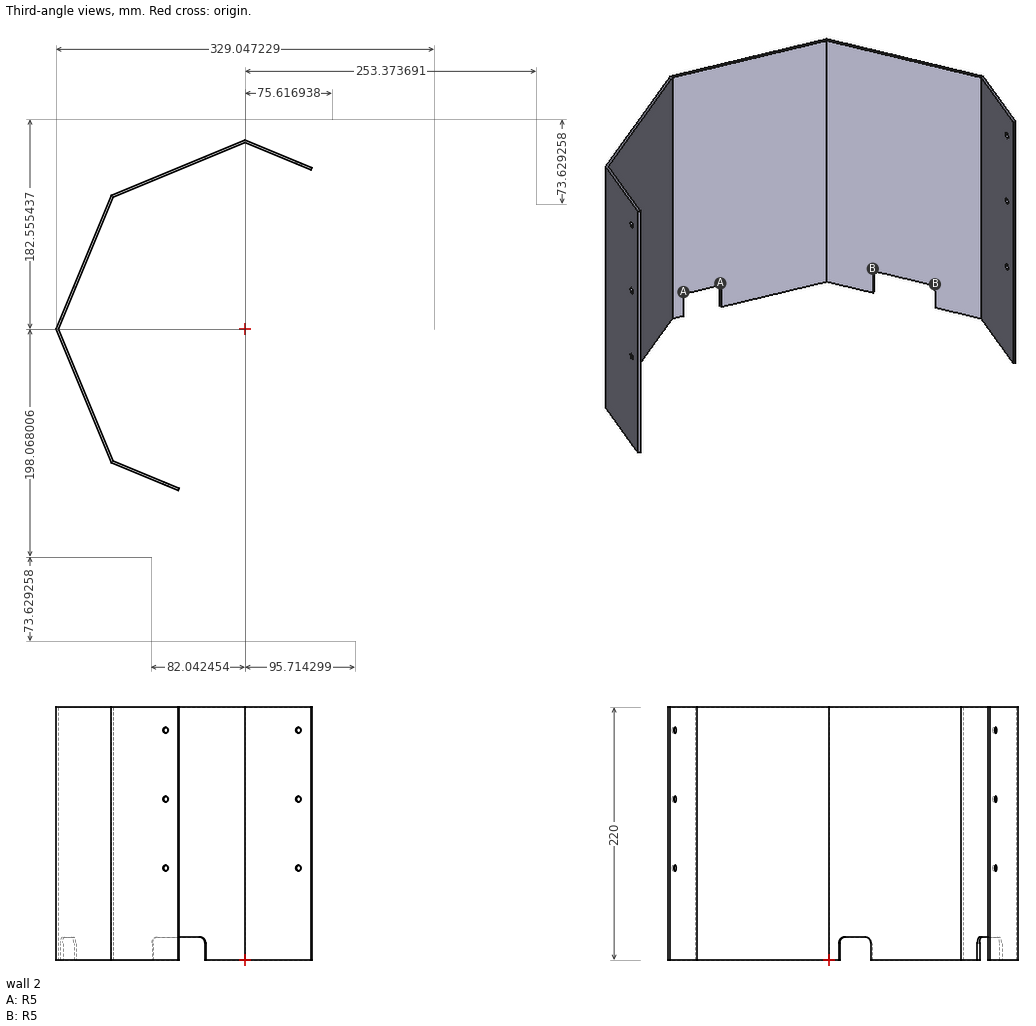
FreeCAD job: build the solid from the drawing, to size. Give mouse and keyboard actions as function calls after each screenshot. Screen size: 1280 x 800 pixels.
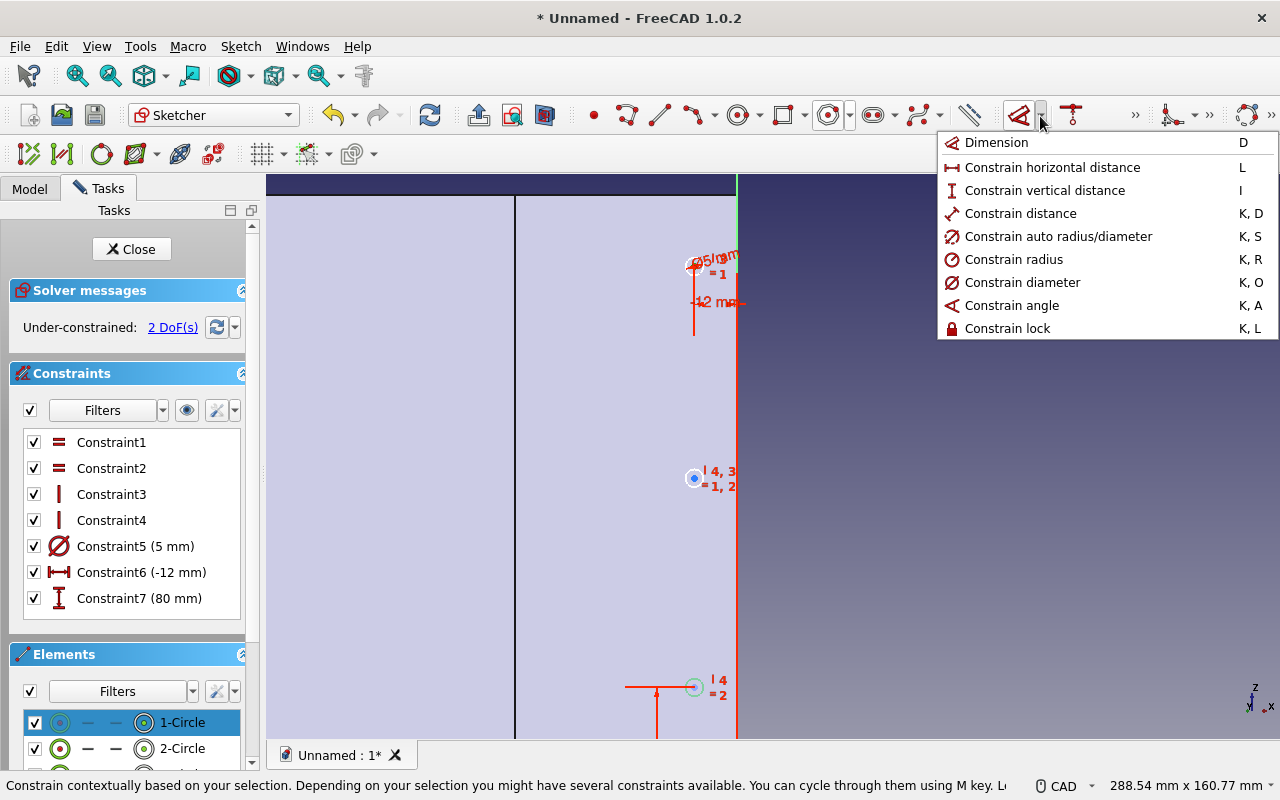
click(1108, 190)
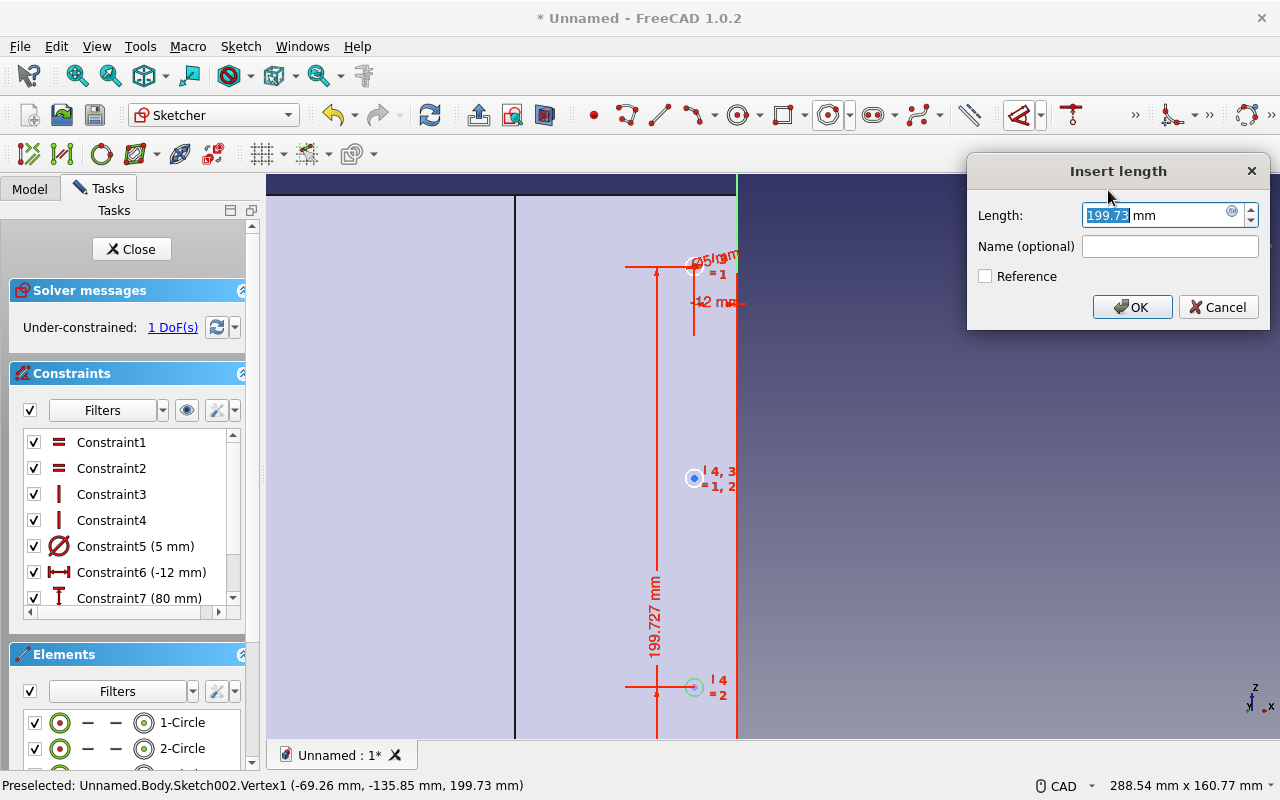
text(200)
key(Return)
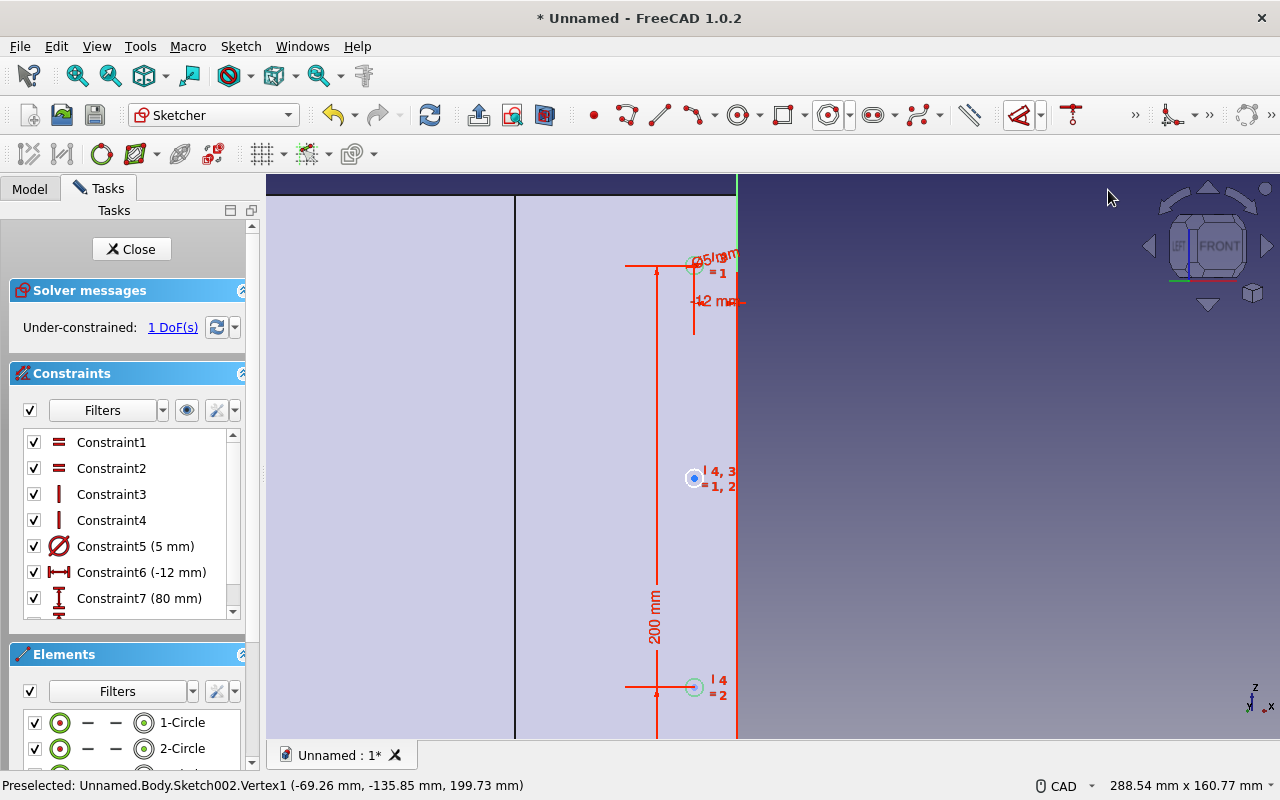
click(694, 478)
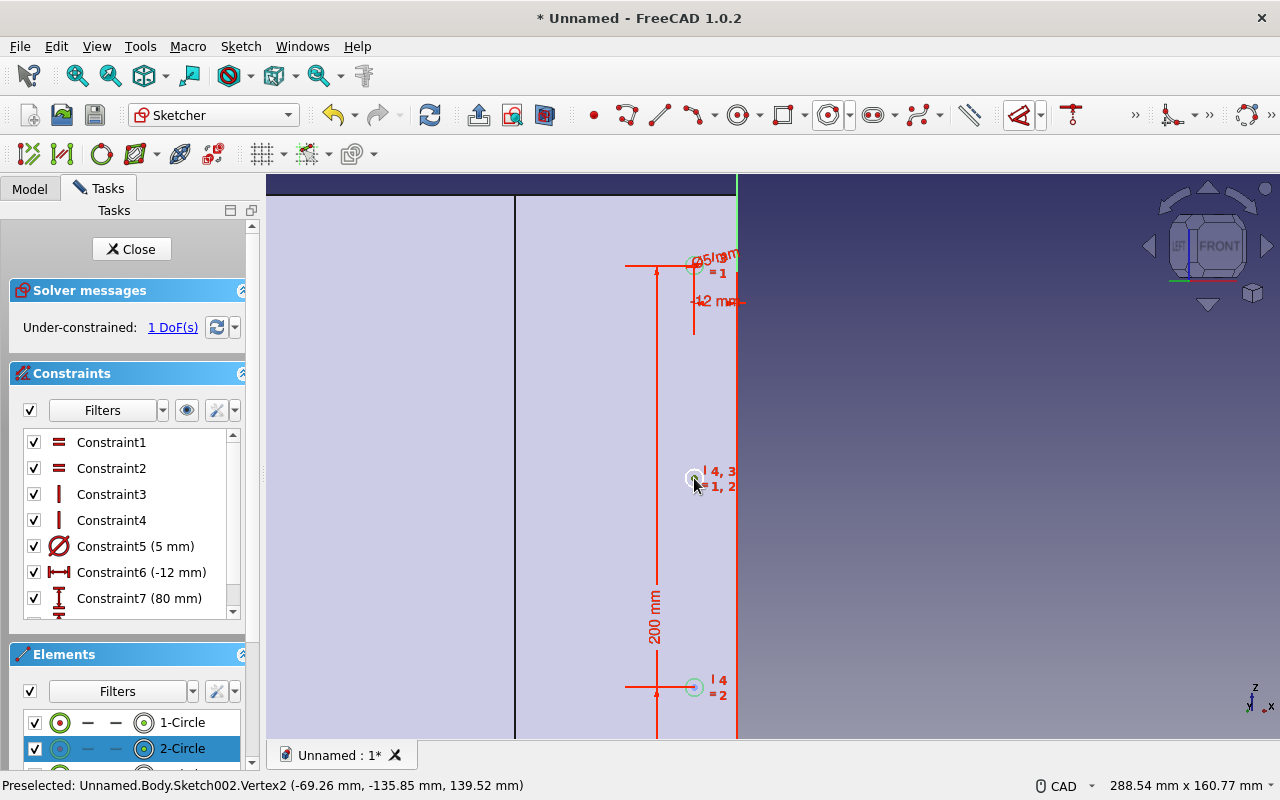
click(1040, 116)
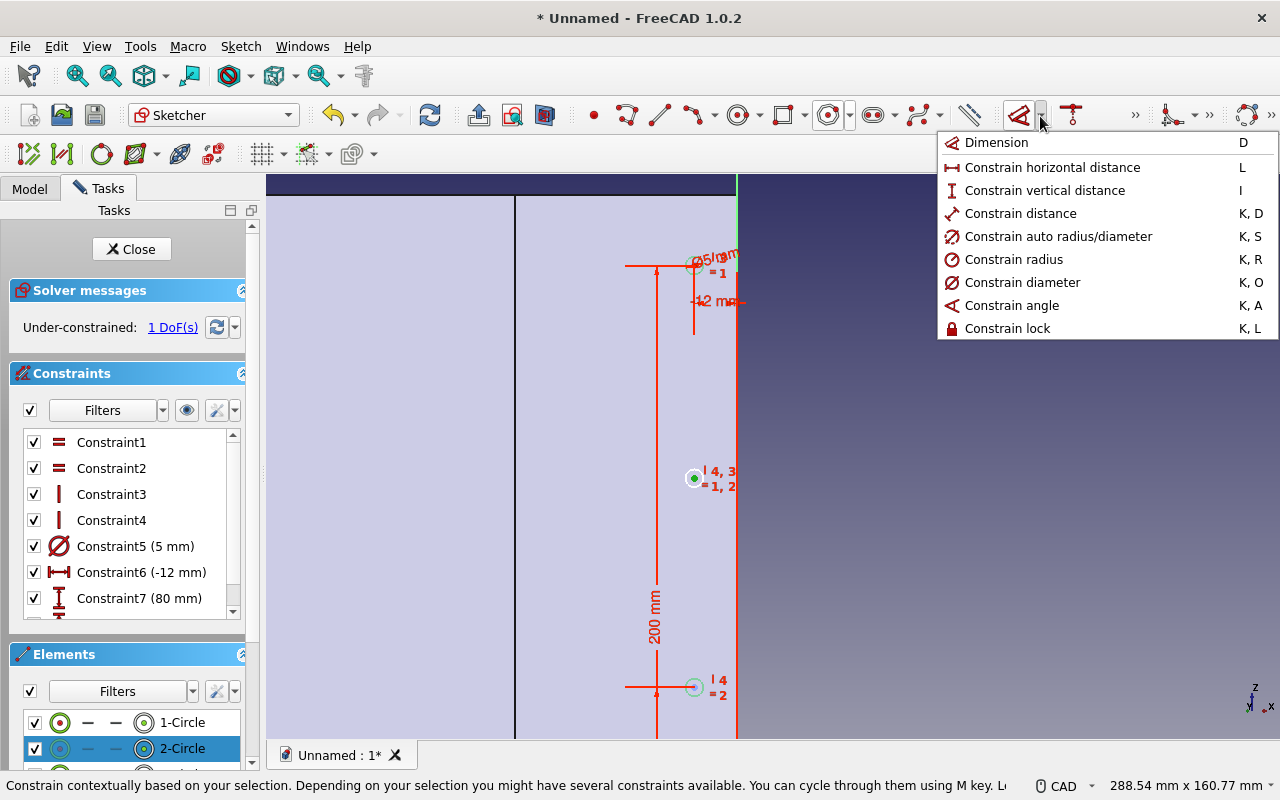
click(1108, 190)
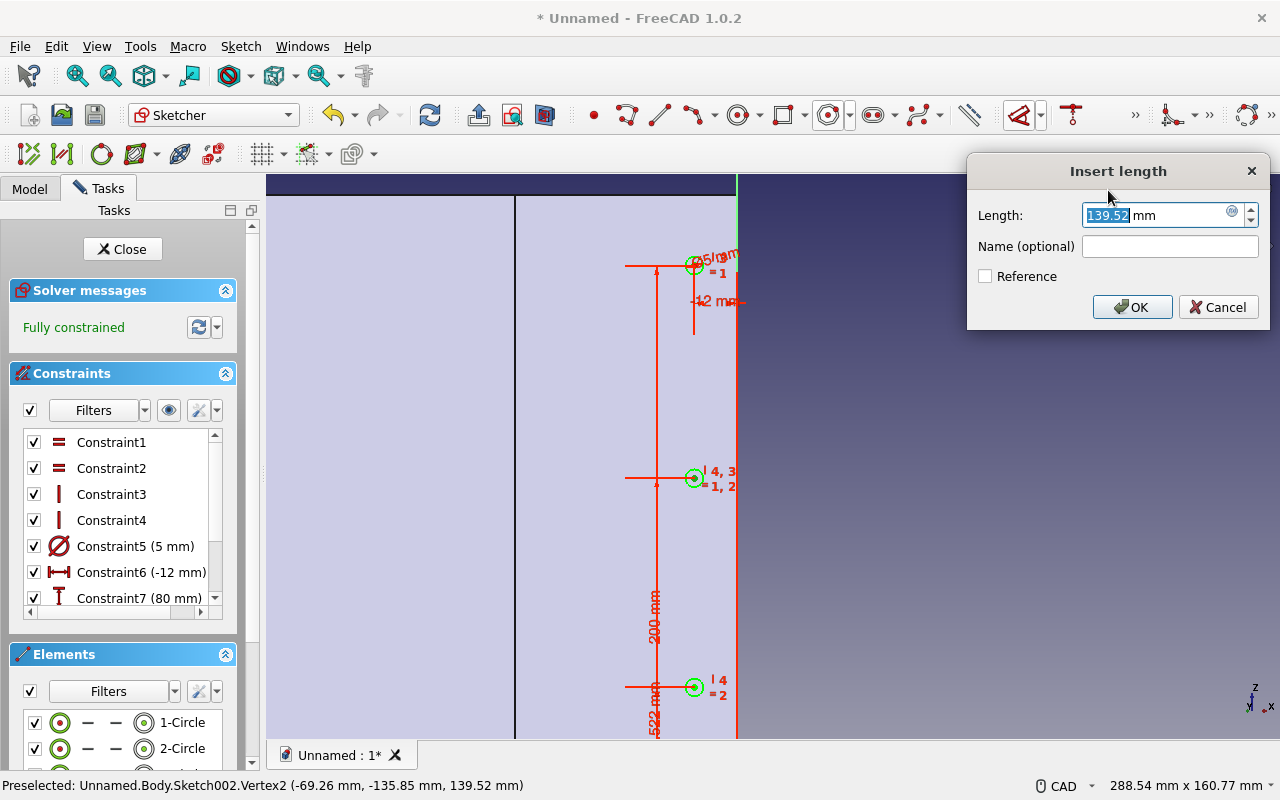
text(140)
key(Return)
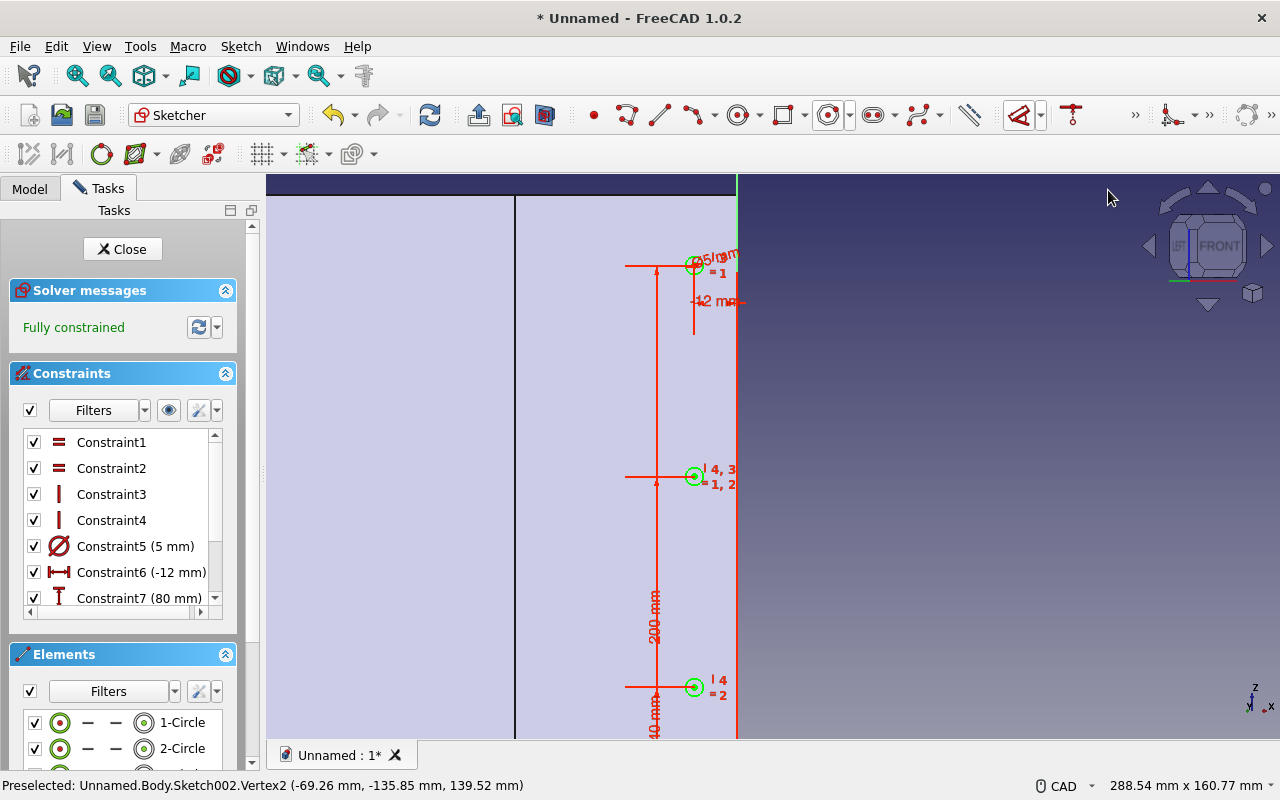
click(123, 249)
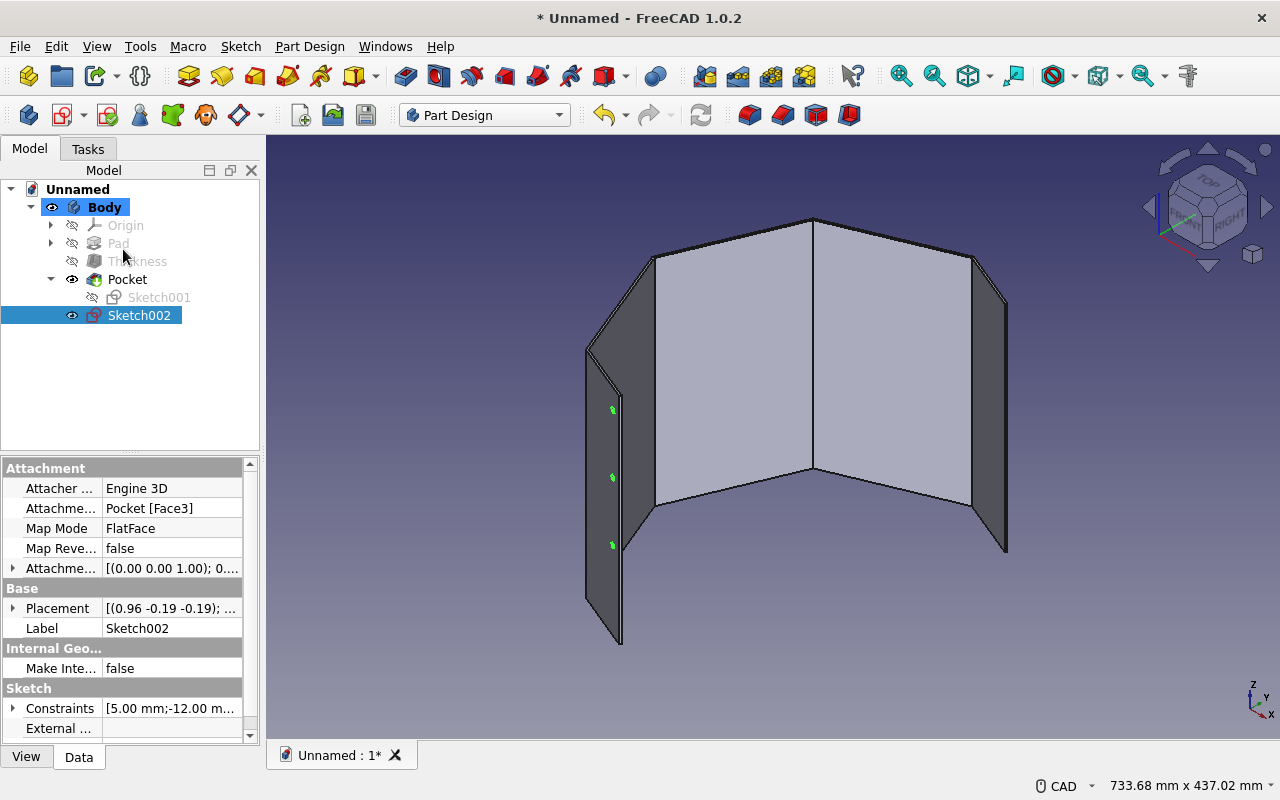
click(406, 76)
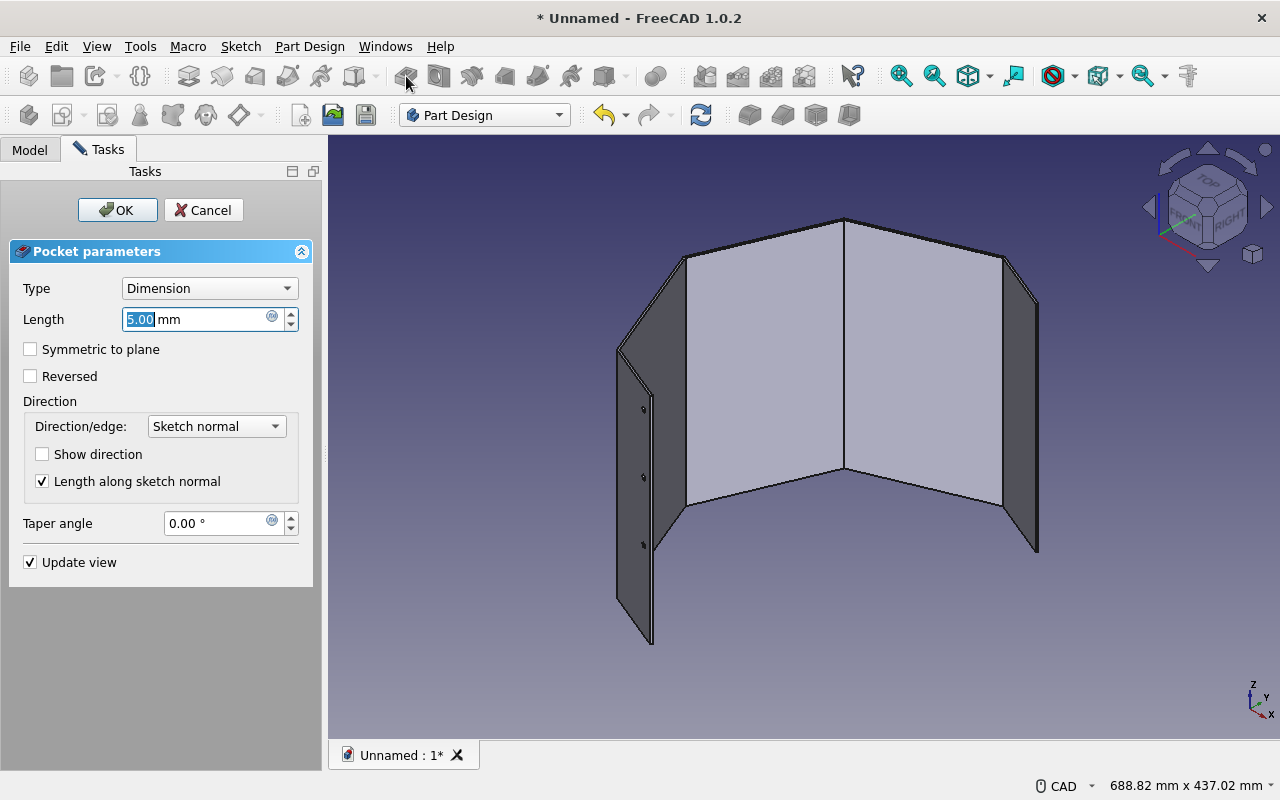
click(210, 288)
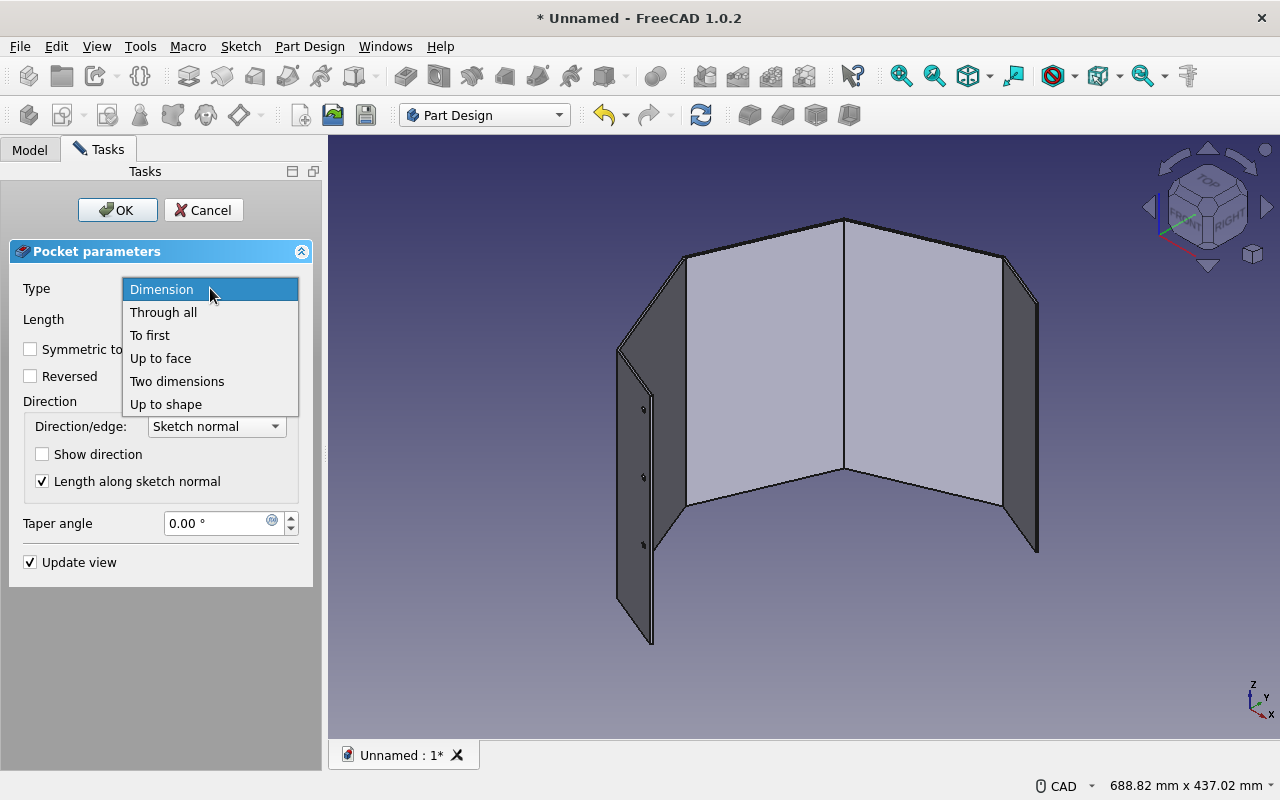
click(208, 312)